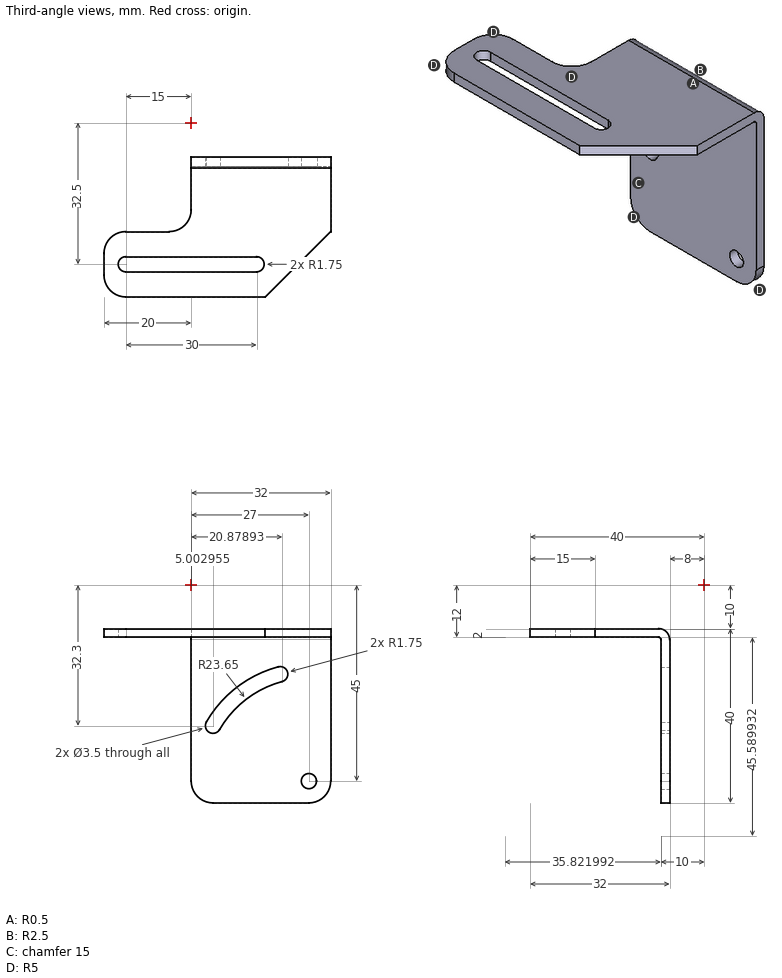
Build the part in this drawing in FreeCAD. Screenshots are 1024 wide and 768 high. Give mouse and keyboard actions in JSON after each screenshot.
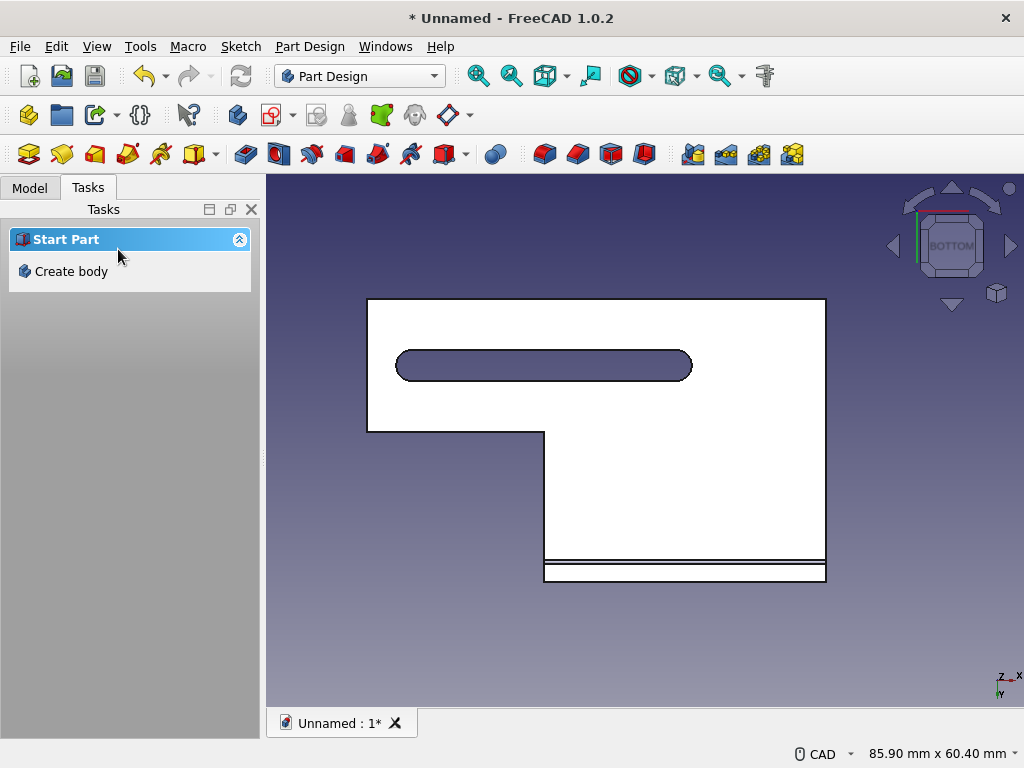
{"action": "scroll", "coordinate": [826, 298], "scroll_direction": "up", "scroll_amount": 5}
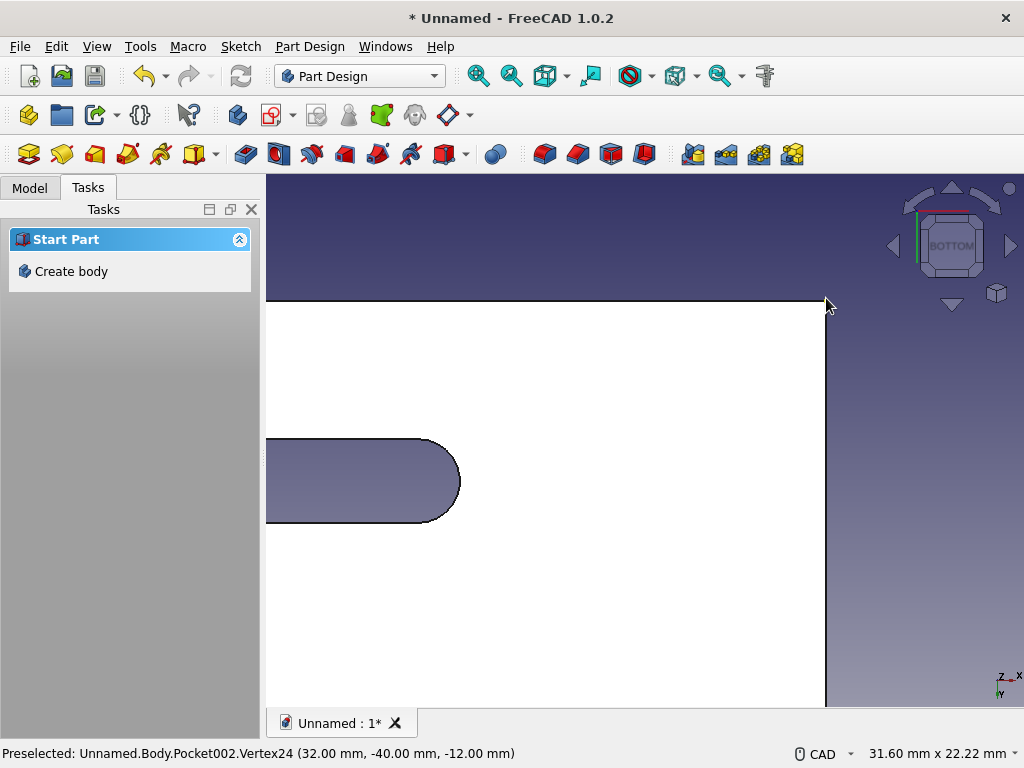
{"action": "key", "text": "v f"}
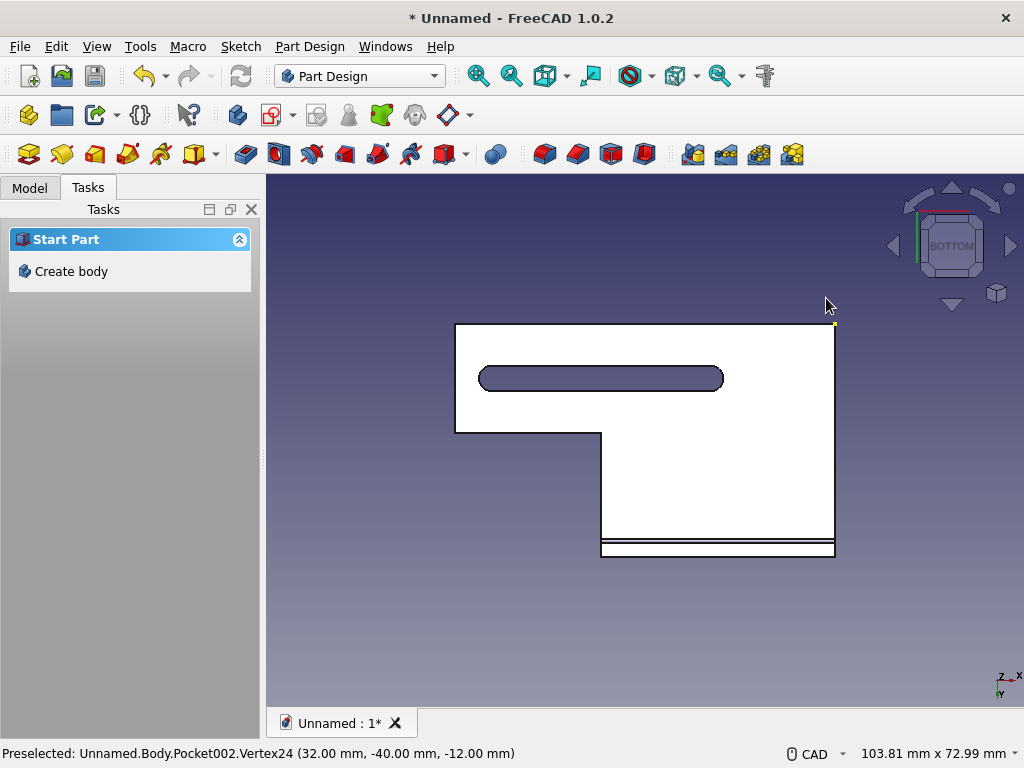
{"action": "key", "text": "0"}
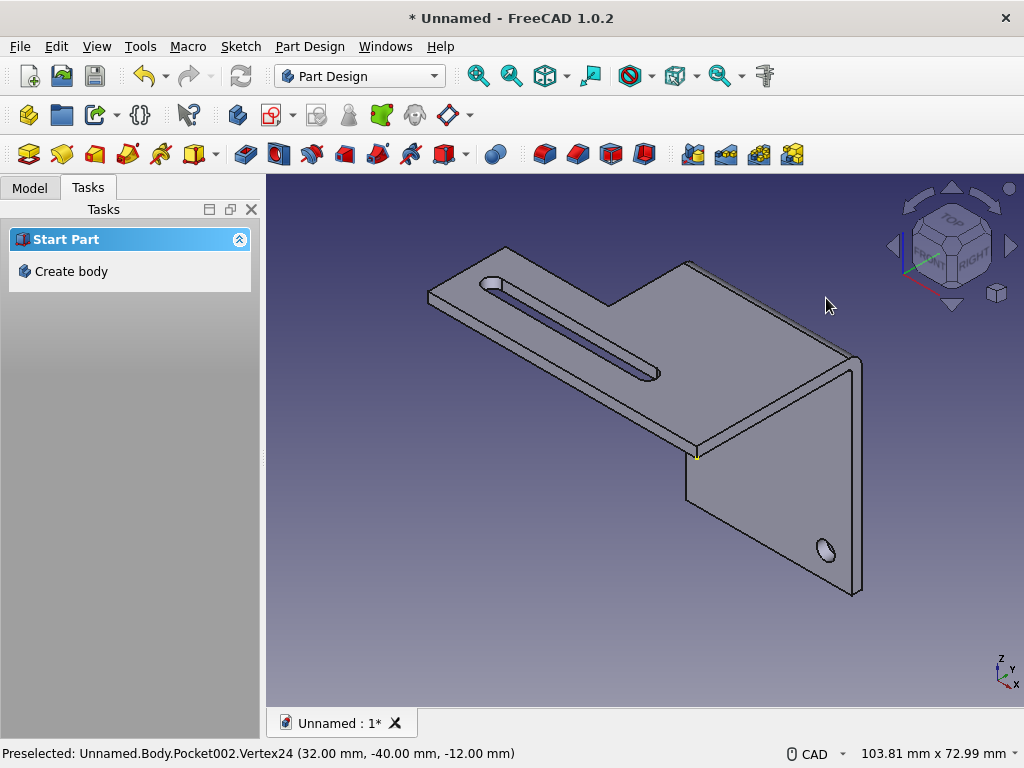
{"action": "left_click", "coordinate": [697, 453]}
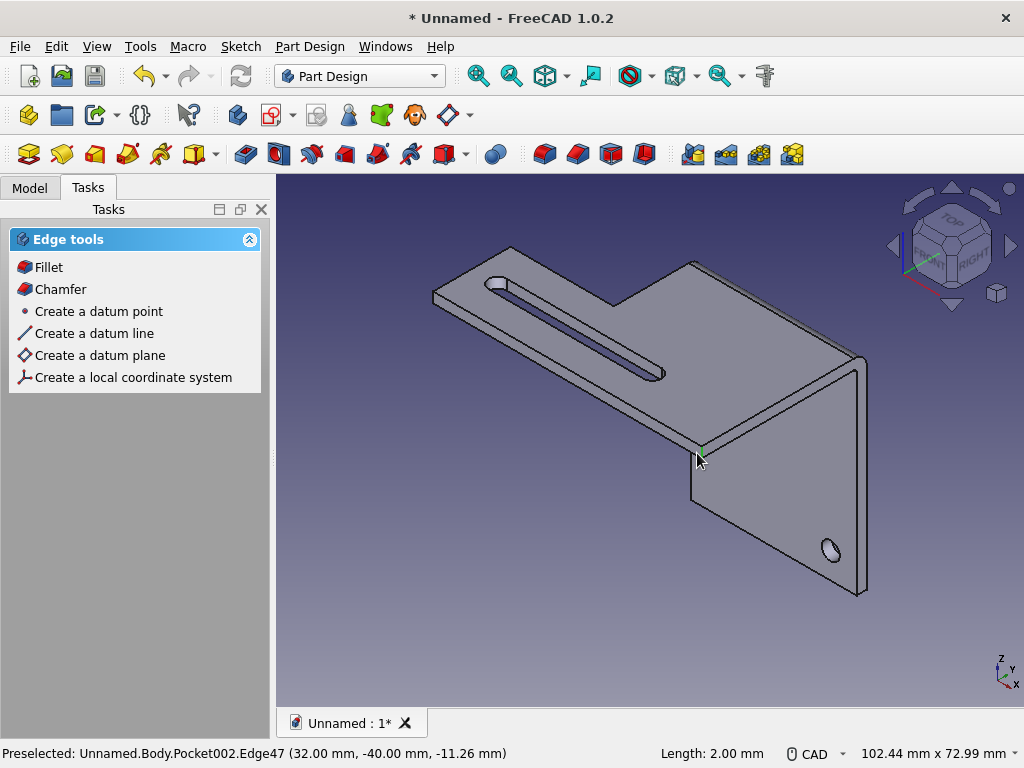
{"action": "left_click", "coordinate": [578, 154]}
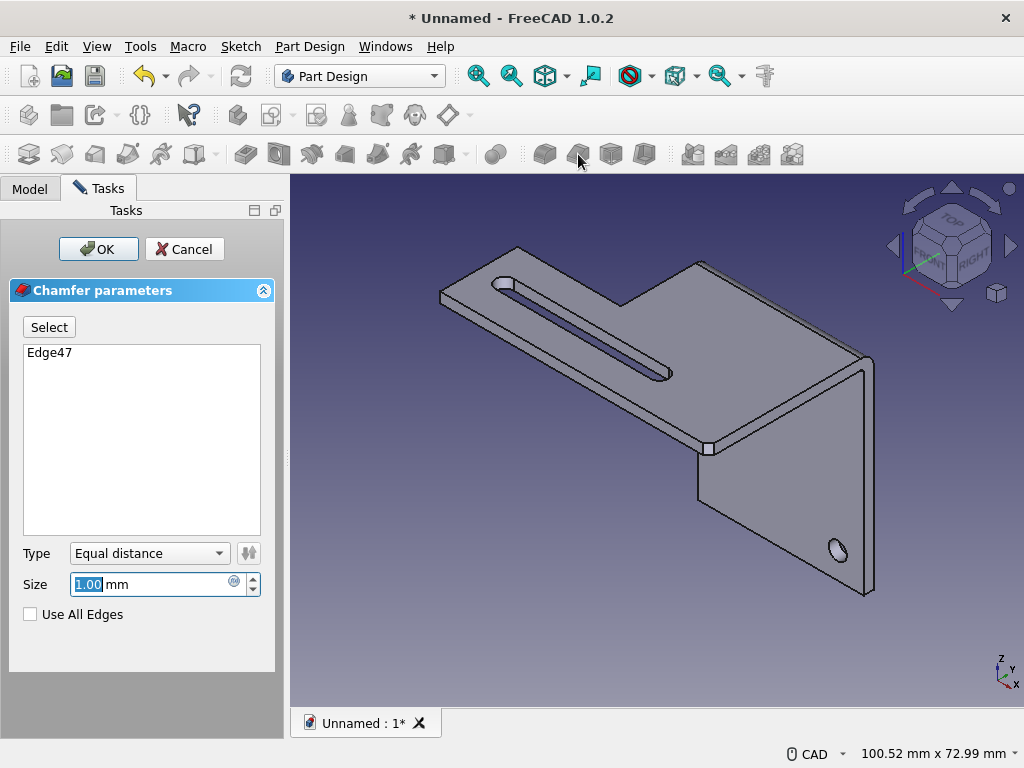
{"action": "type", "text": "15"}
{"action": "key", "text": "Tab"}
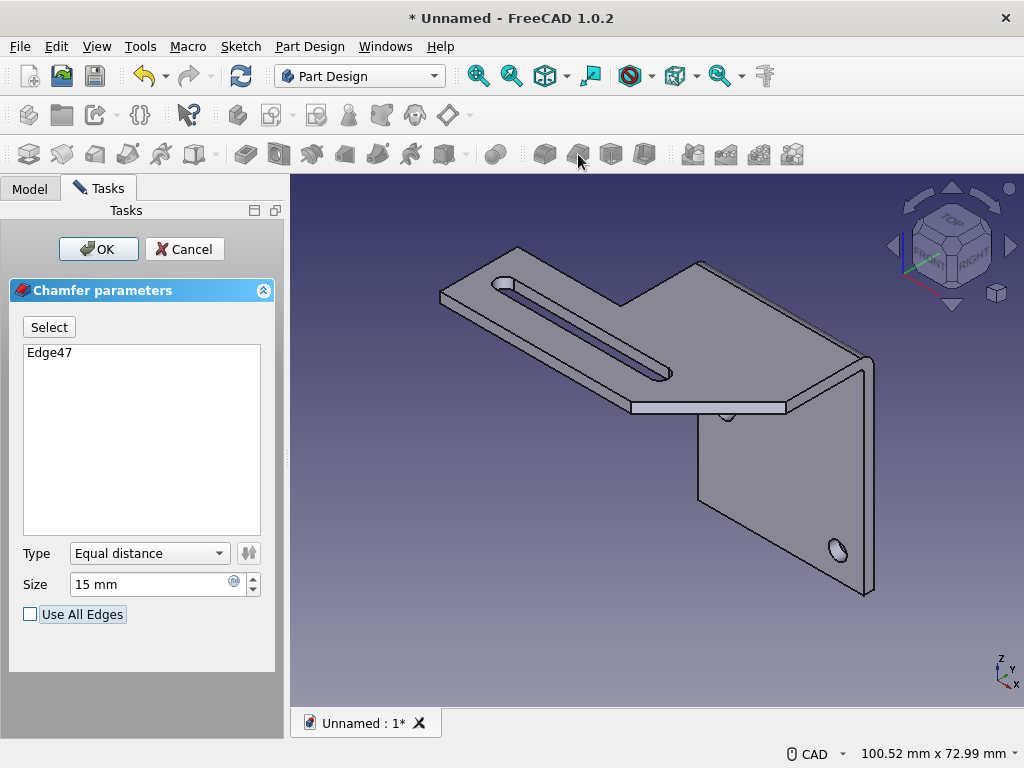
{"action": "left_click", "coordinate": [99, 249]}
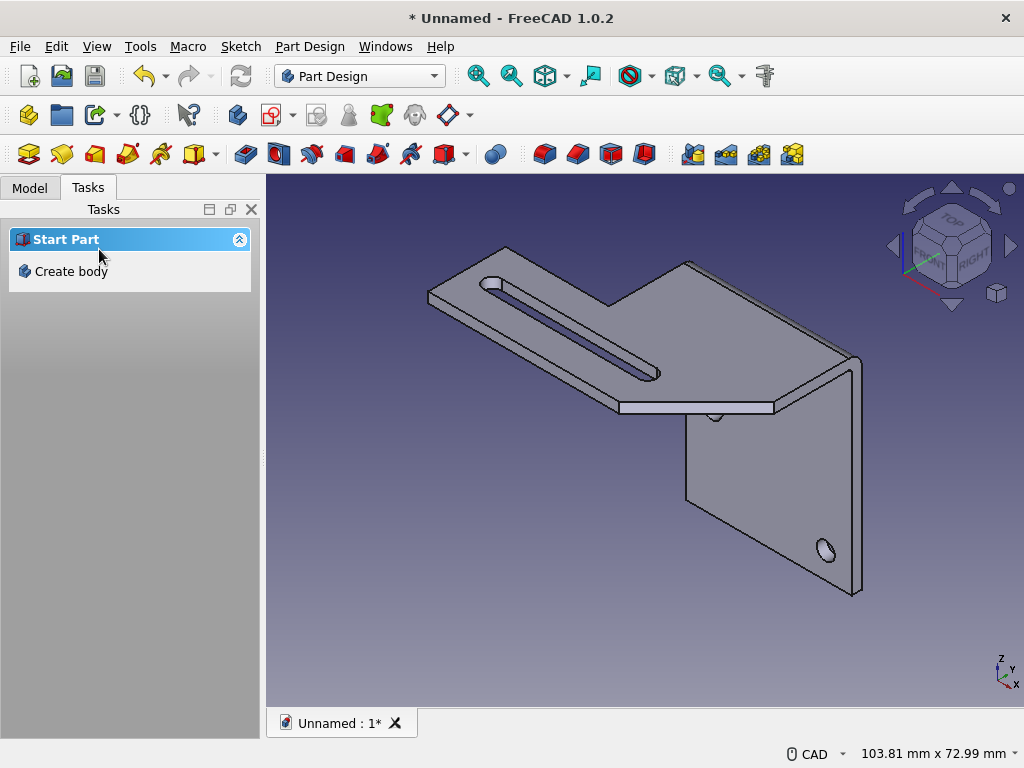
{"action": "scroll", "coordinate": [428, 296], "scroll_direction": "up", "scroll_amount": 6}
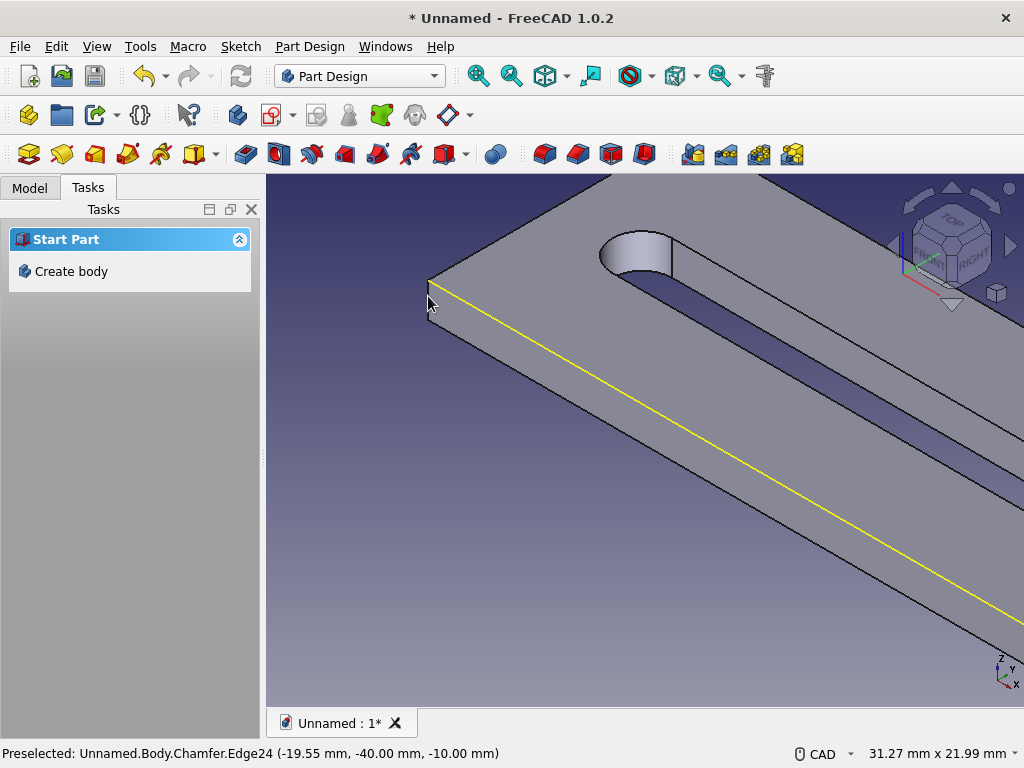
{"action": "key", "text": "v f"}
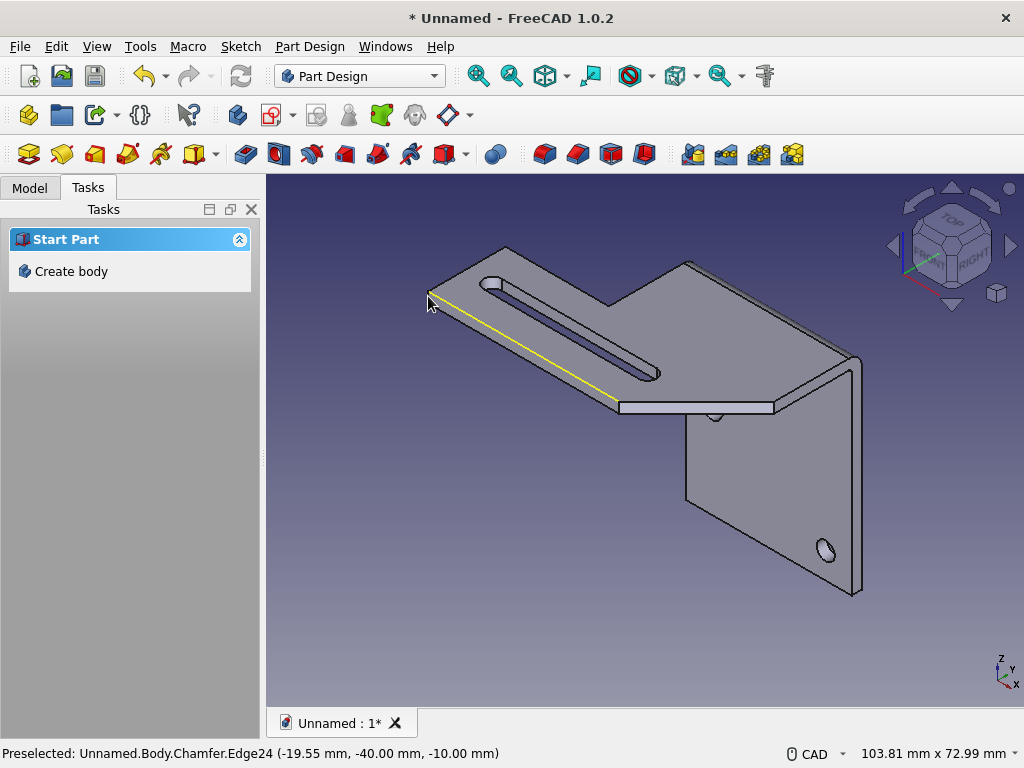
{"action": "key", "text": "2"}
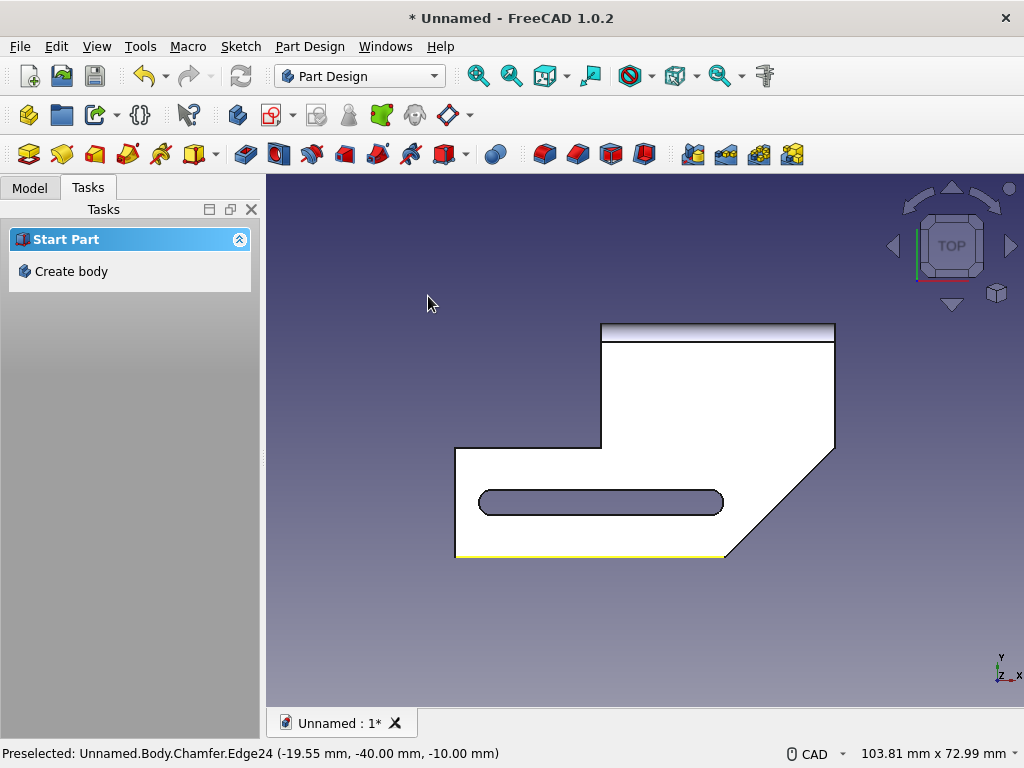
{"action": "scroll", "coordinate": [455, 556], "scroll_direction": "up", "scroll_amount": 6}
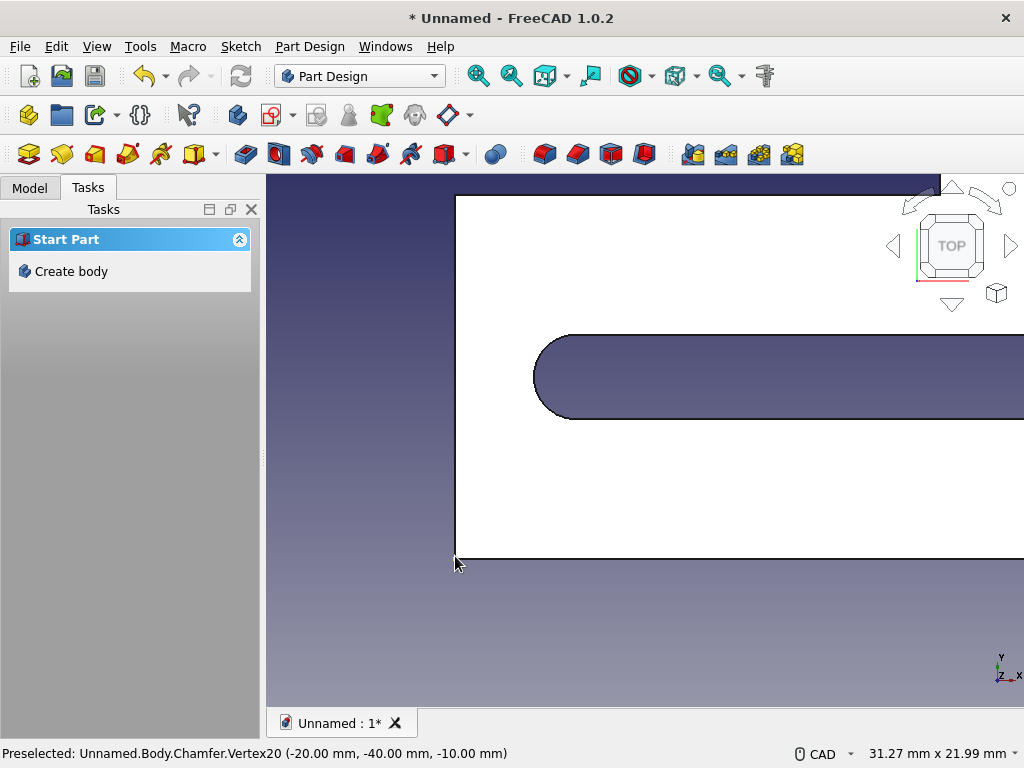
{"action": "key", "text": "v f"}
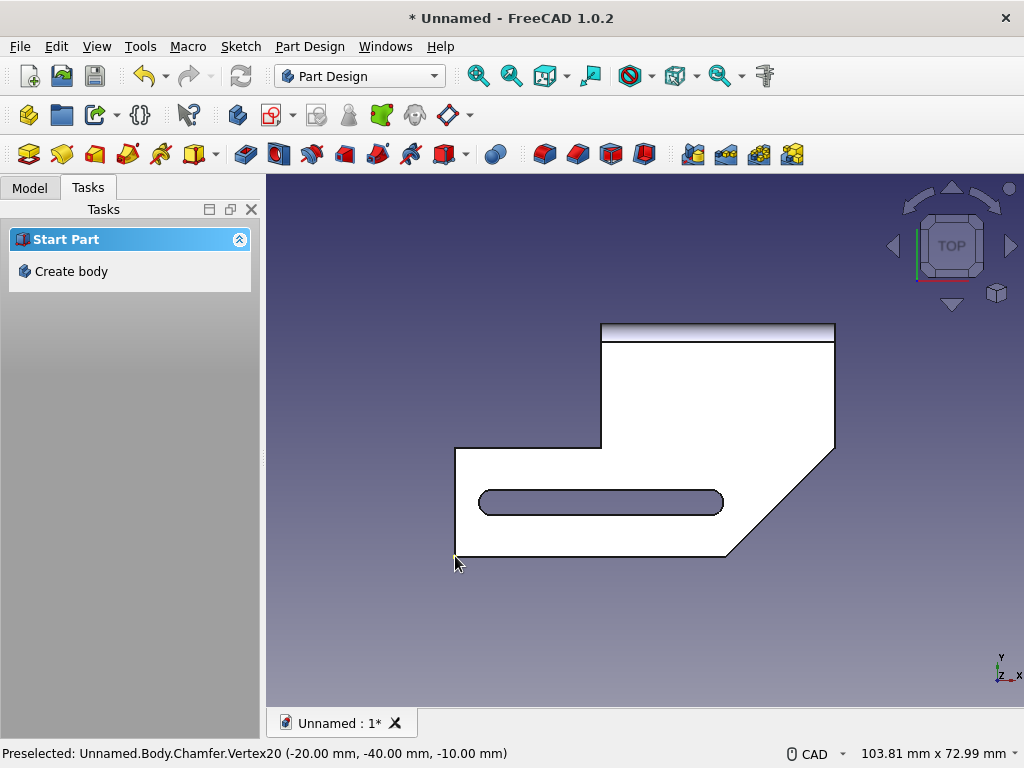
{"action": "key", "text": "0"}